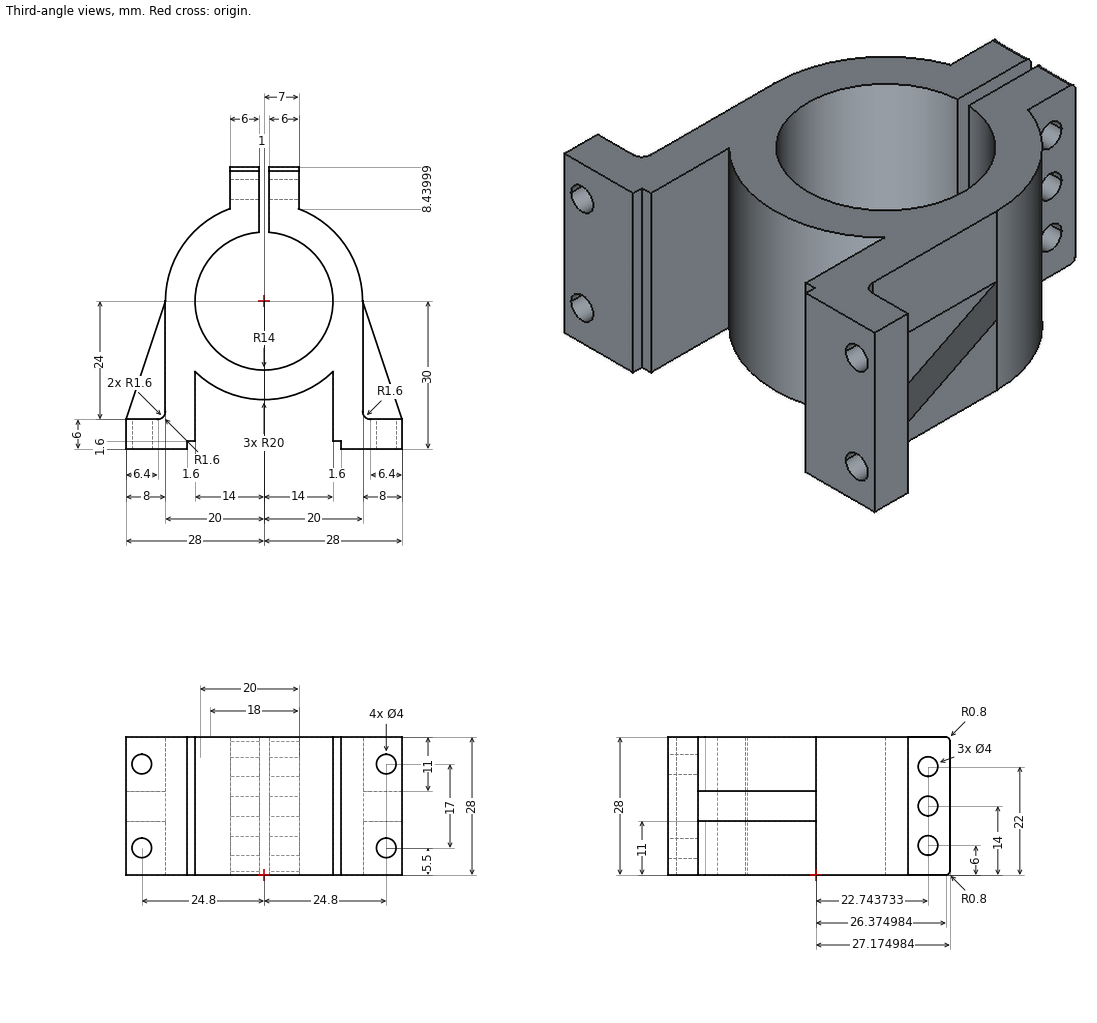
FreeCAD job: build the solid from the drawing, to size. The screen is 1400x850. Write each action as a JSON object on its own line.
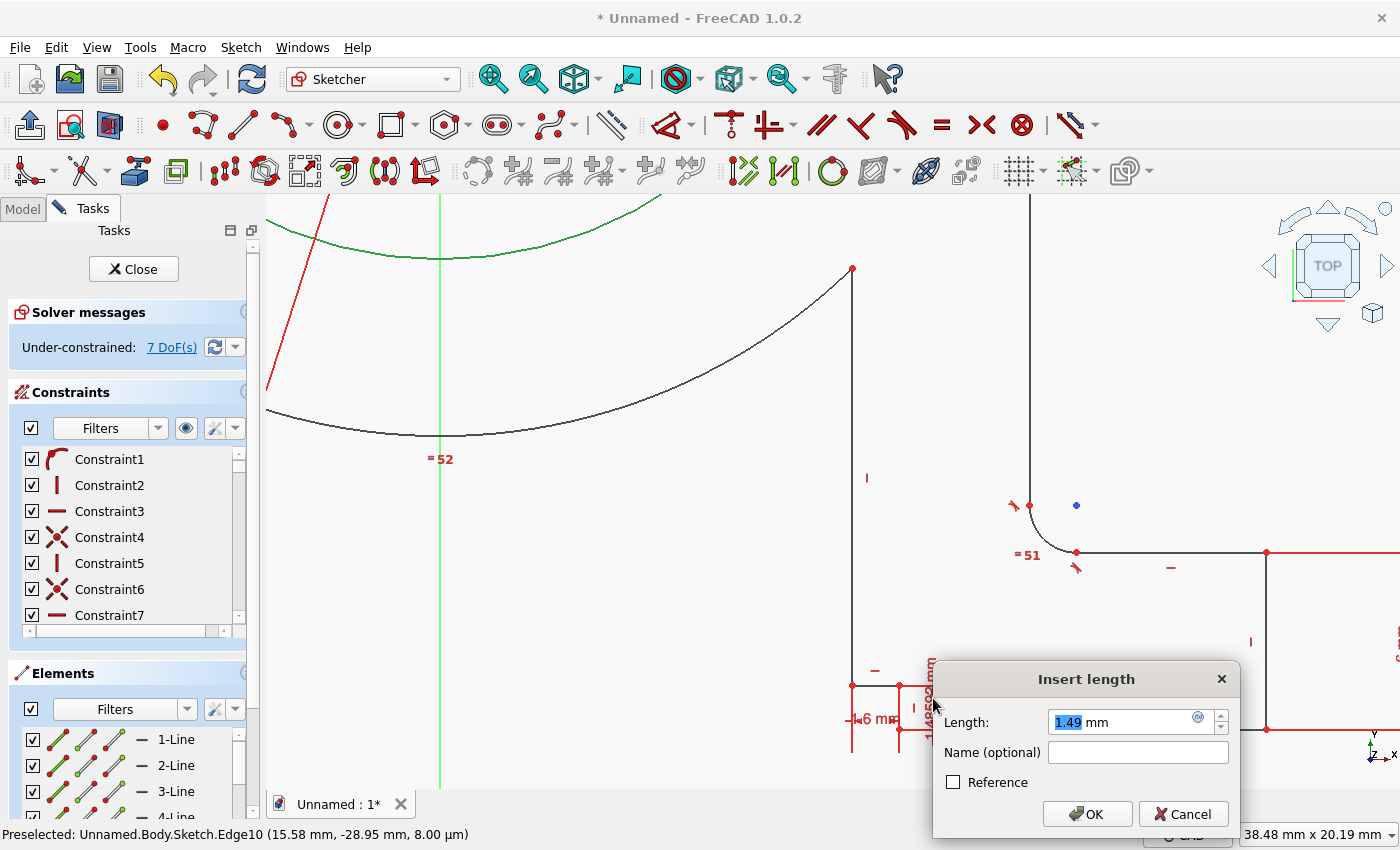
{"action": "type", "text": "1.6"}
{"action": "key", "text": "Return"}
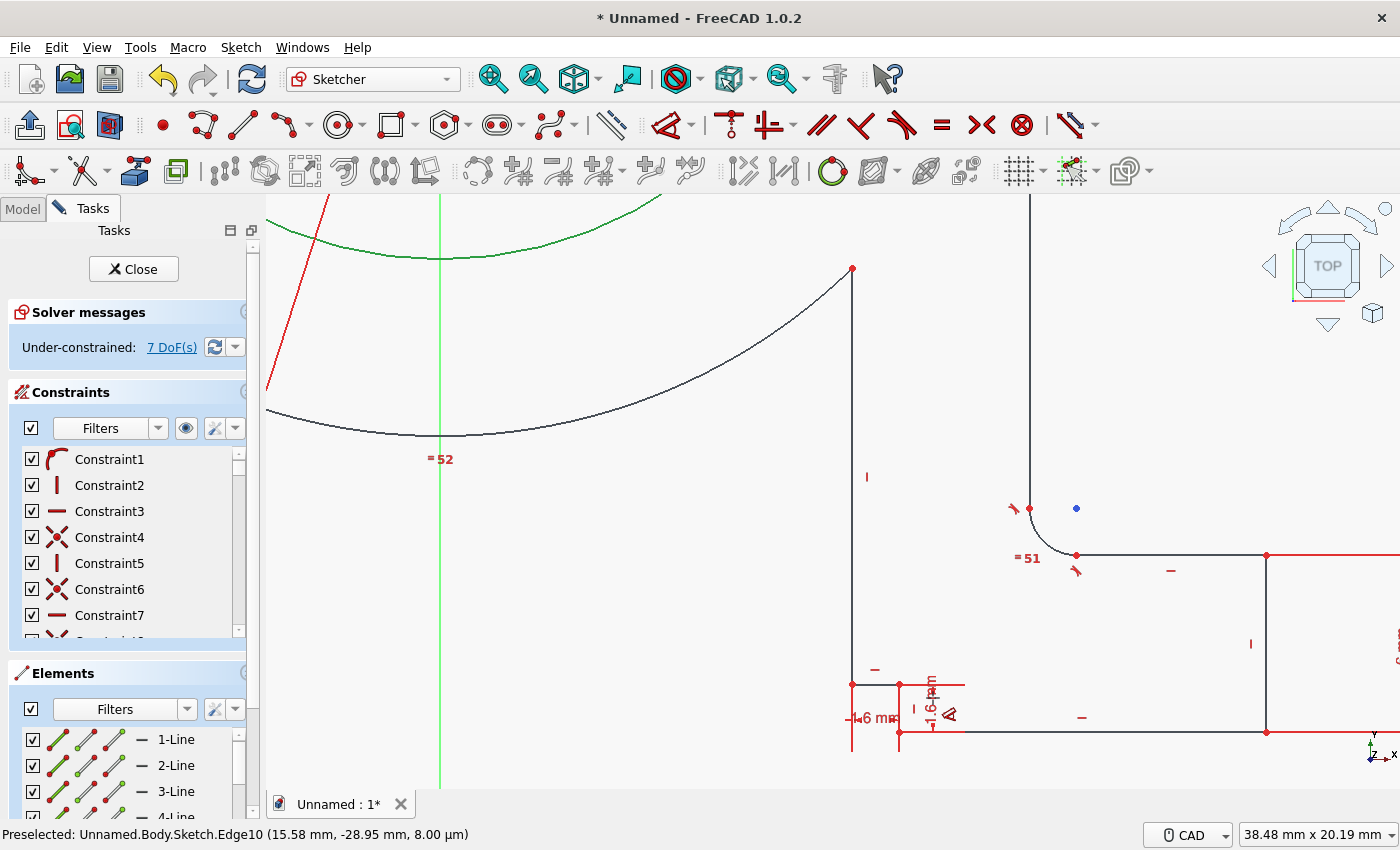
{"action": "scroll", "coordinate": [871, 689], "scroll_direction": "down", "scroll_amount": 7}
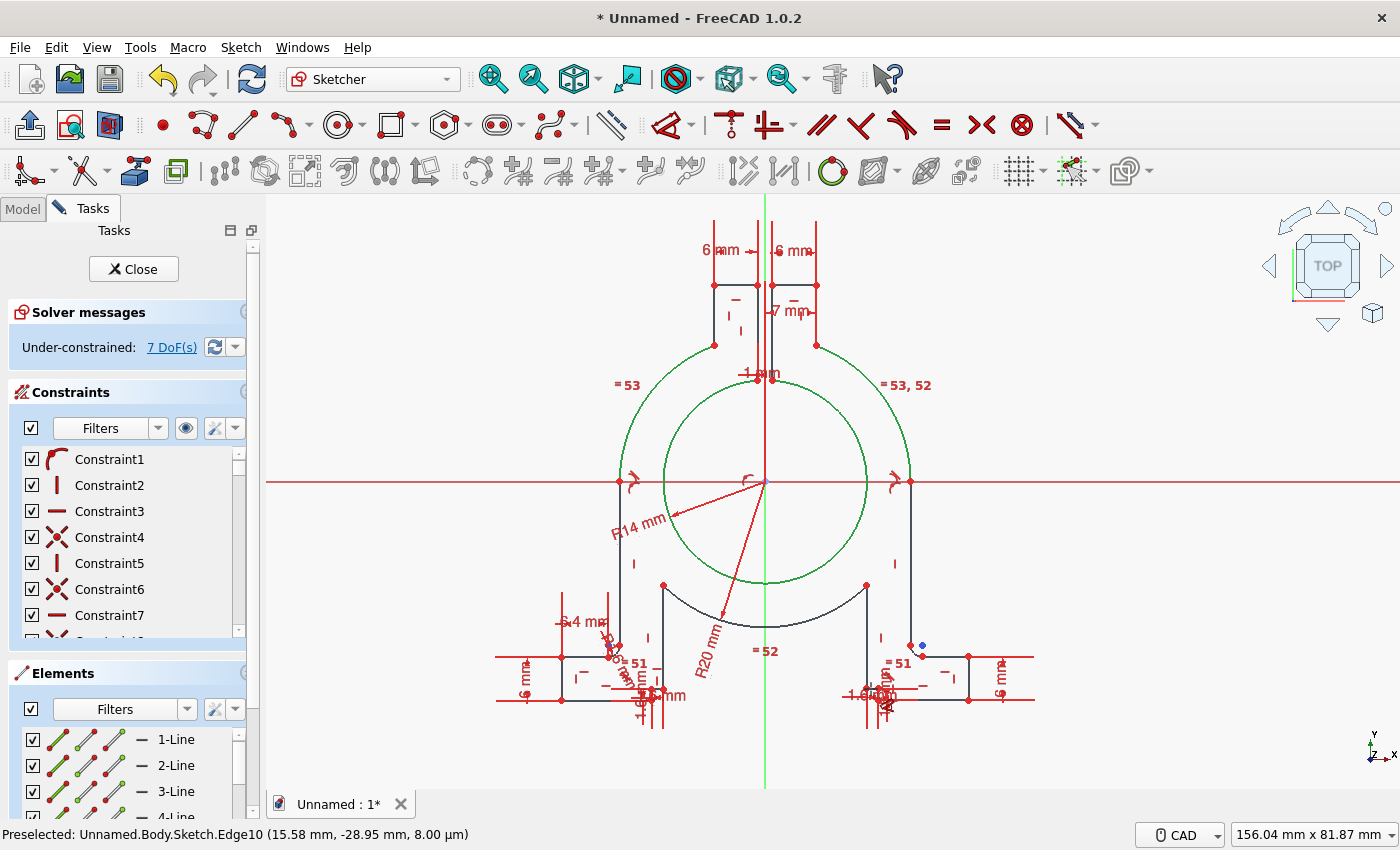
{"action": "left_click", "coordinate": [955, 657]}
{"action": "left_click", "coordinate": [946, 623]}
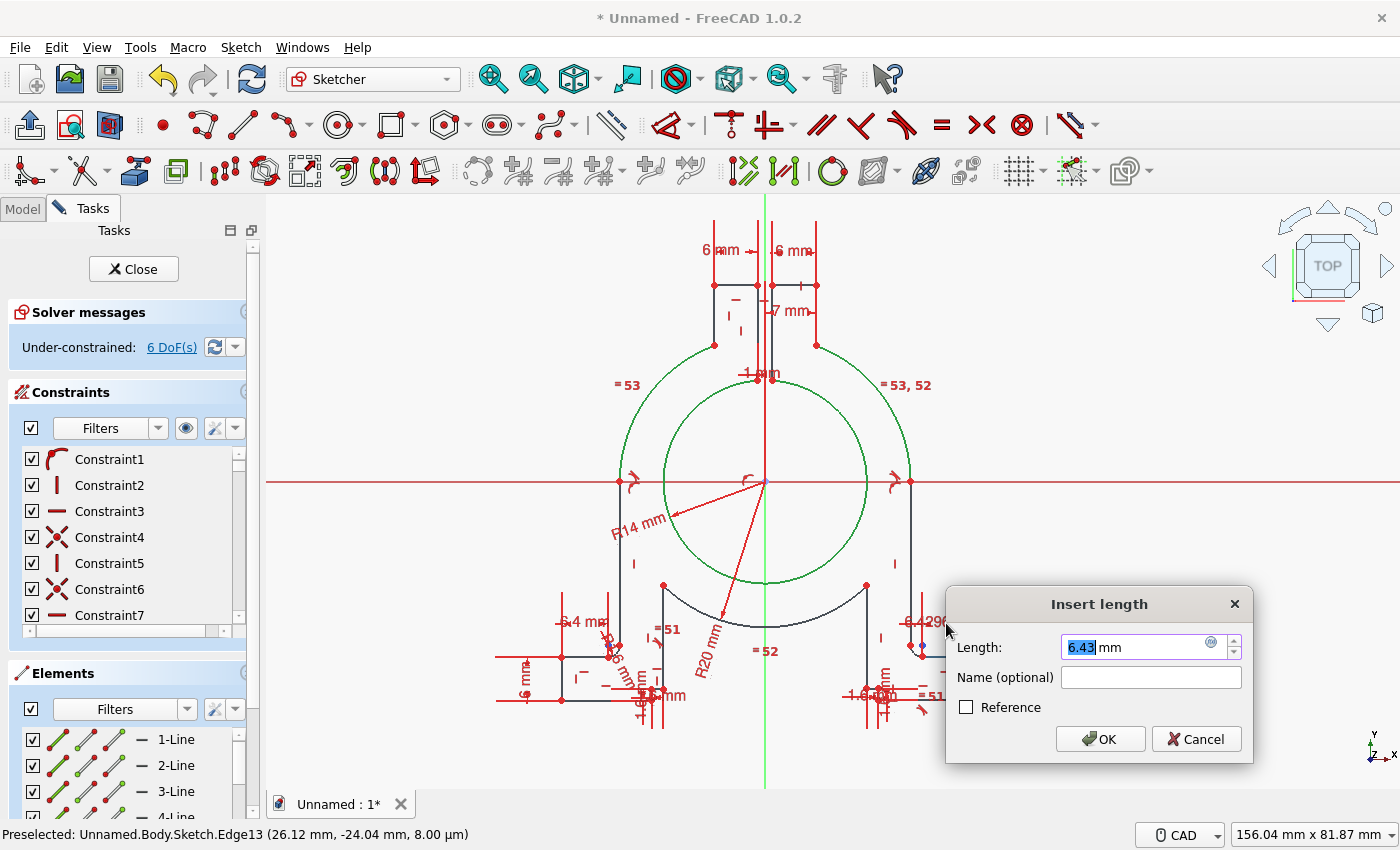
{"action": "type", "text": "6.4"}
{"action": "key", "text": "Return"}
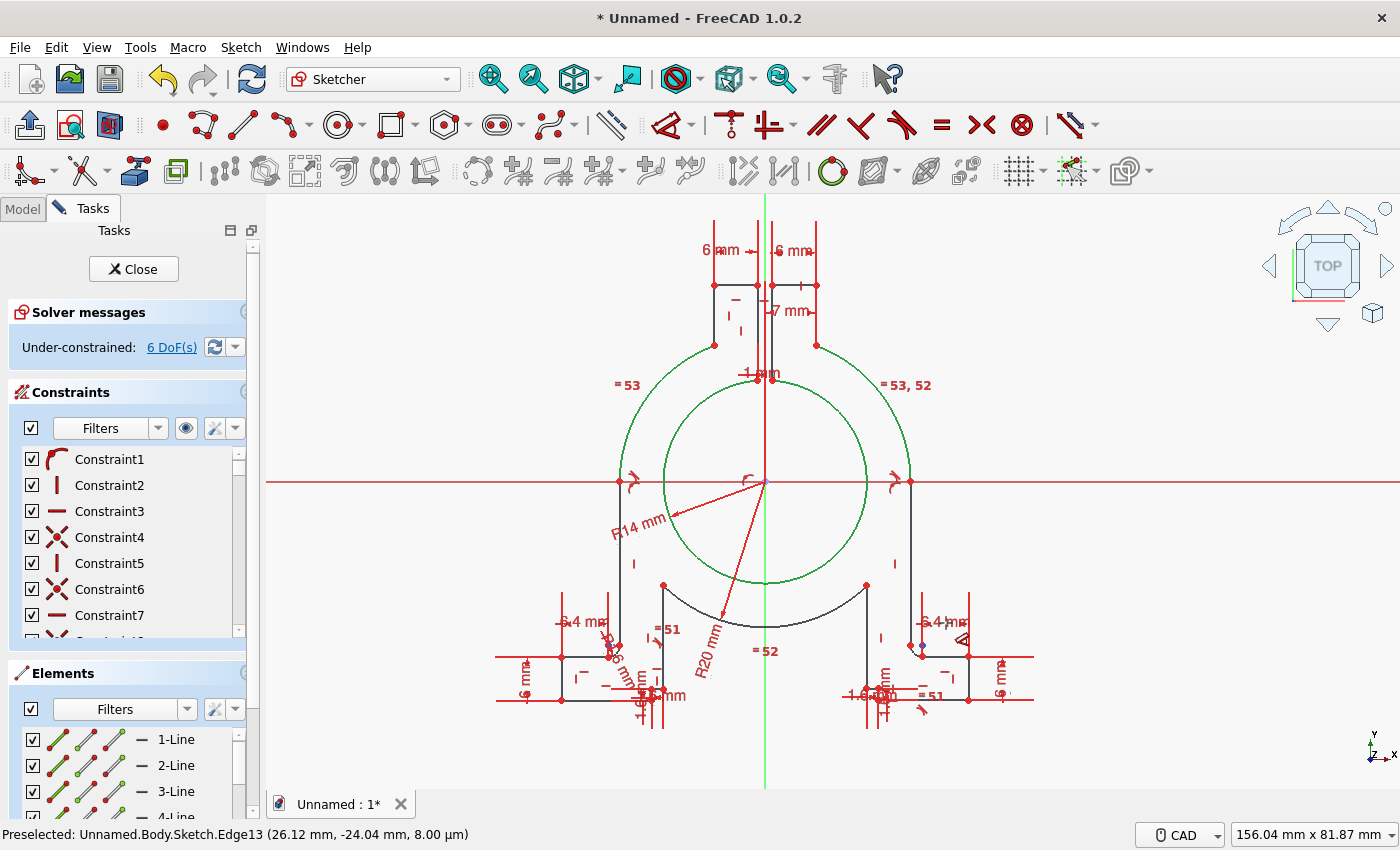
{"action": "left_click", "coordinate": [608, 657]}
{"action": "left_click", "coordinate": [574, 569]}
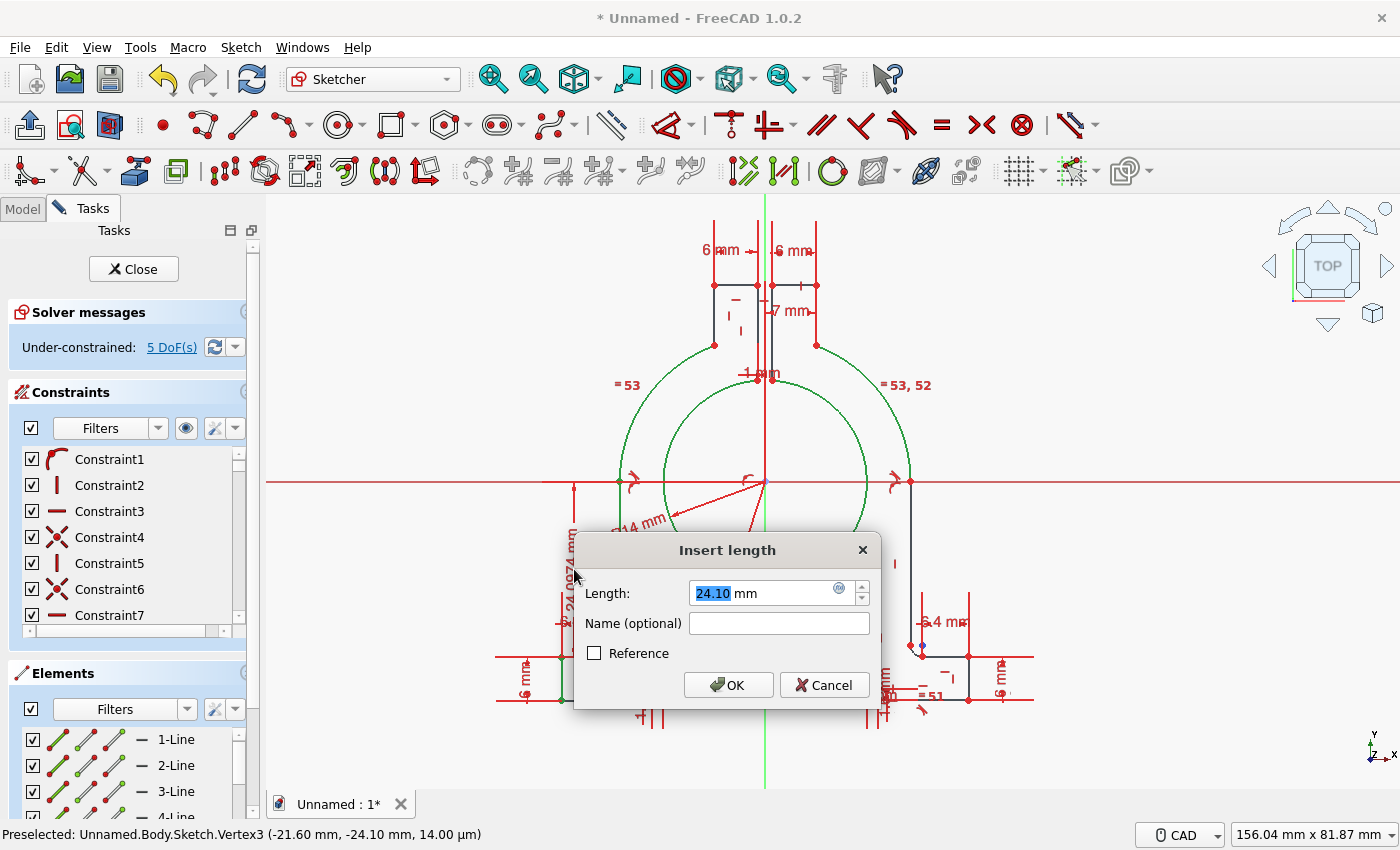
{"action": "type", "text": "24"}
{"action": "key", "text": "Return"}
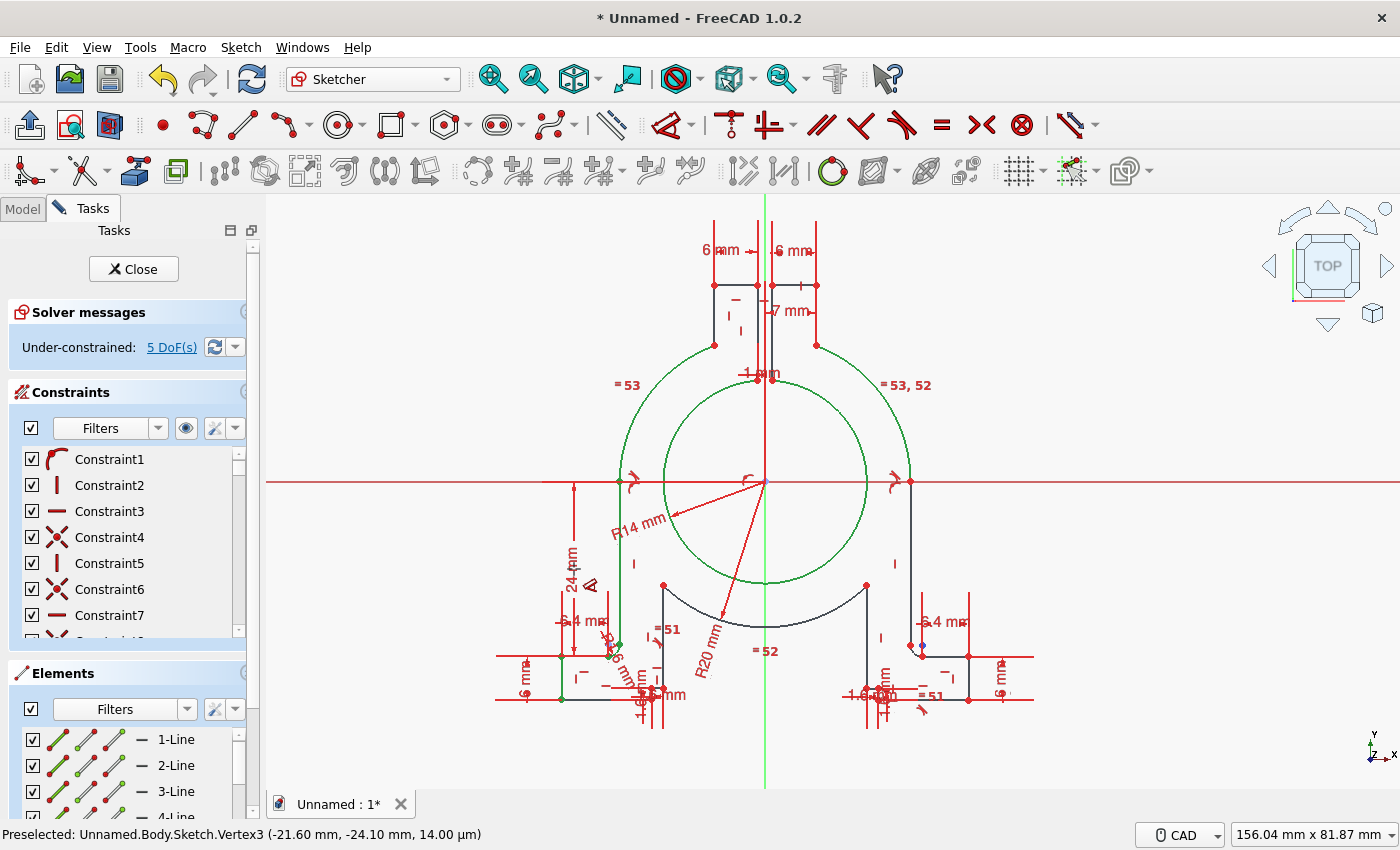
{"action": "left_click", "coordinate": [663, 688]}
{"action": "left_click", "coordinate": [714, 722]}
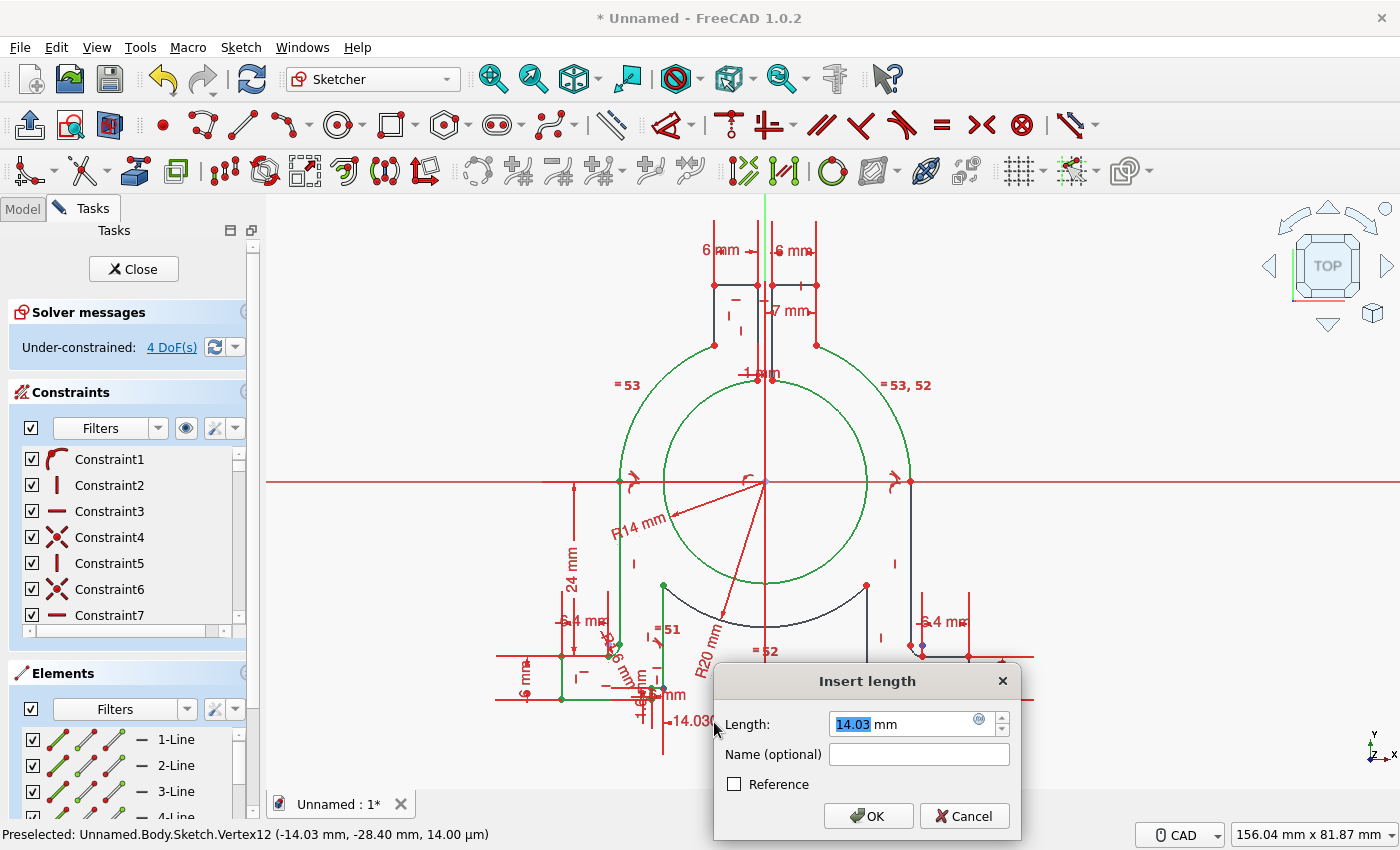
{"action": "type", "text": "14"}
{"action": "key", "text": "Return"}